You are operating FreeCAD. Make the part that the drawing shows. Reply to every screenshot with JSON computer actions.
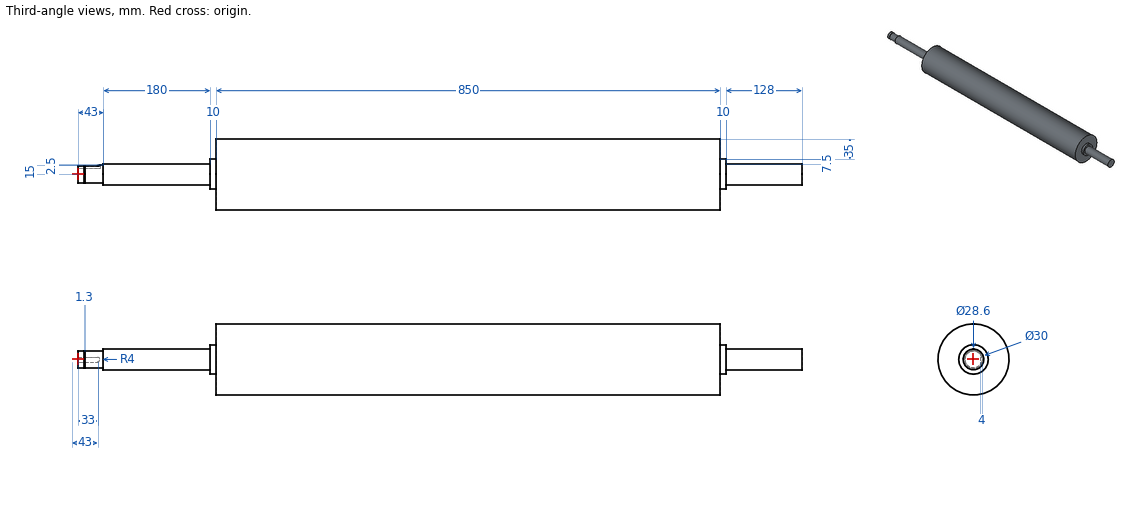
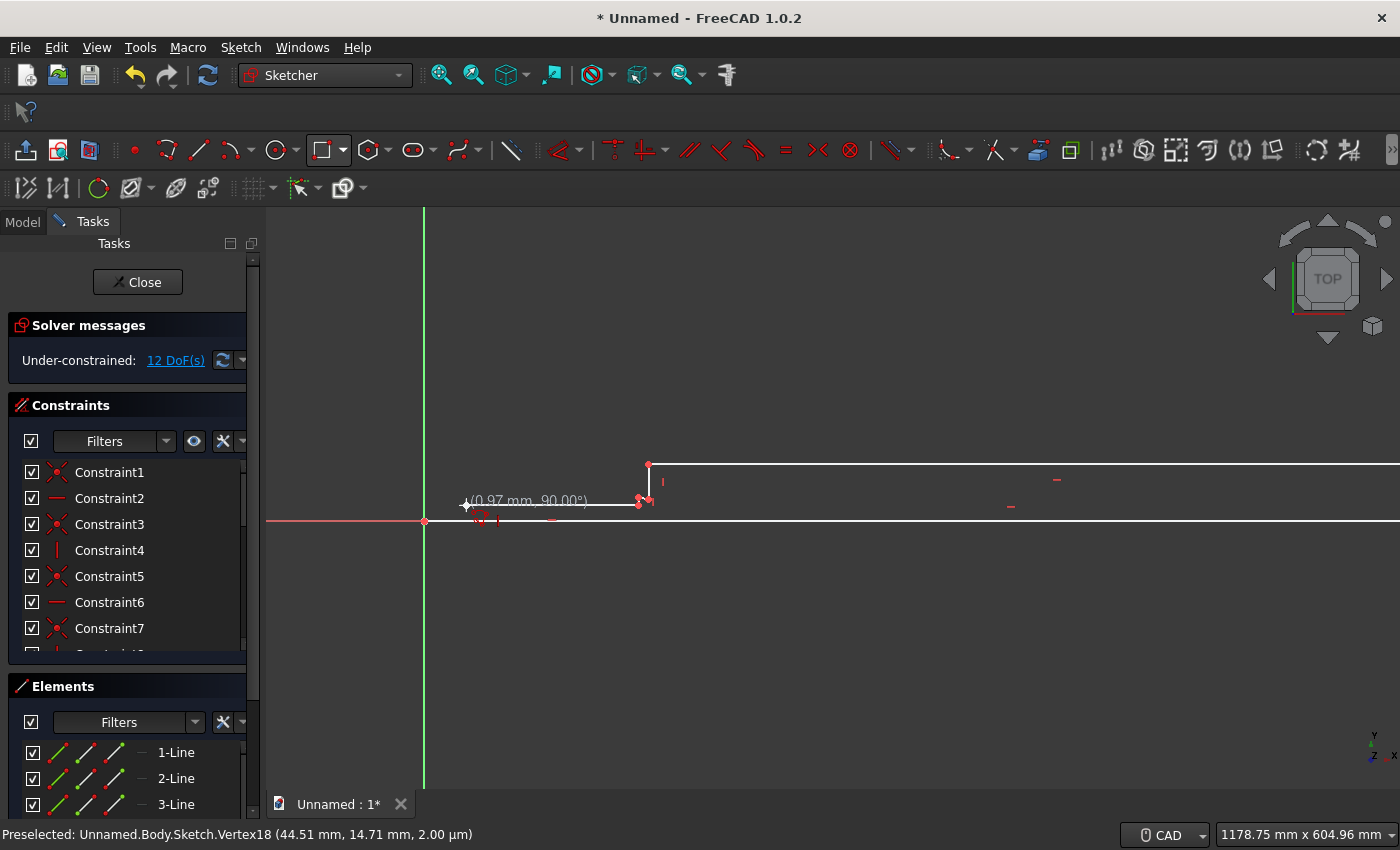
{"action": "scroll", "coordinate": [466, 507], "scroll_direction": "up", "scroll_amount": 10}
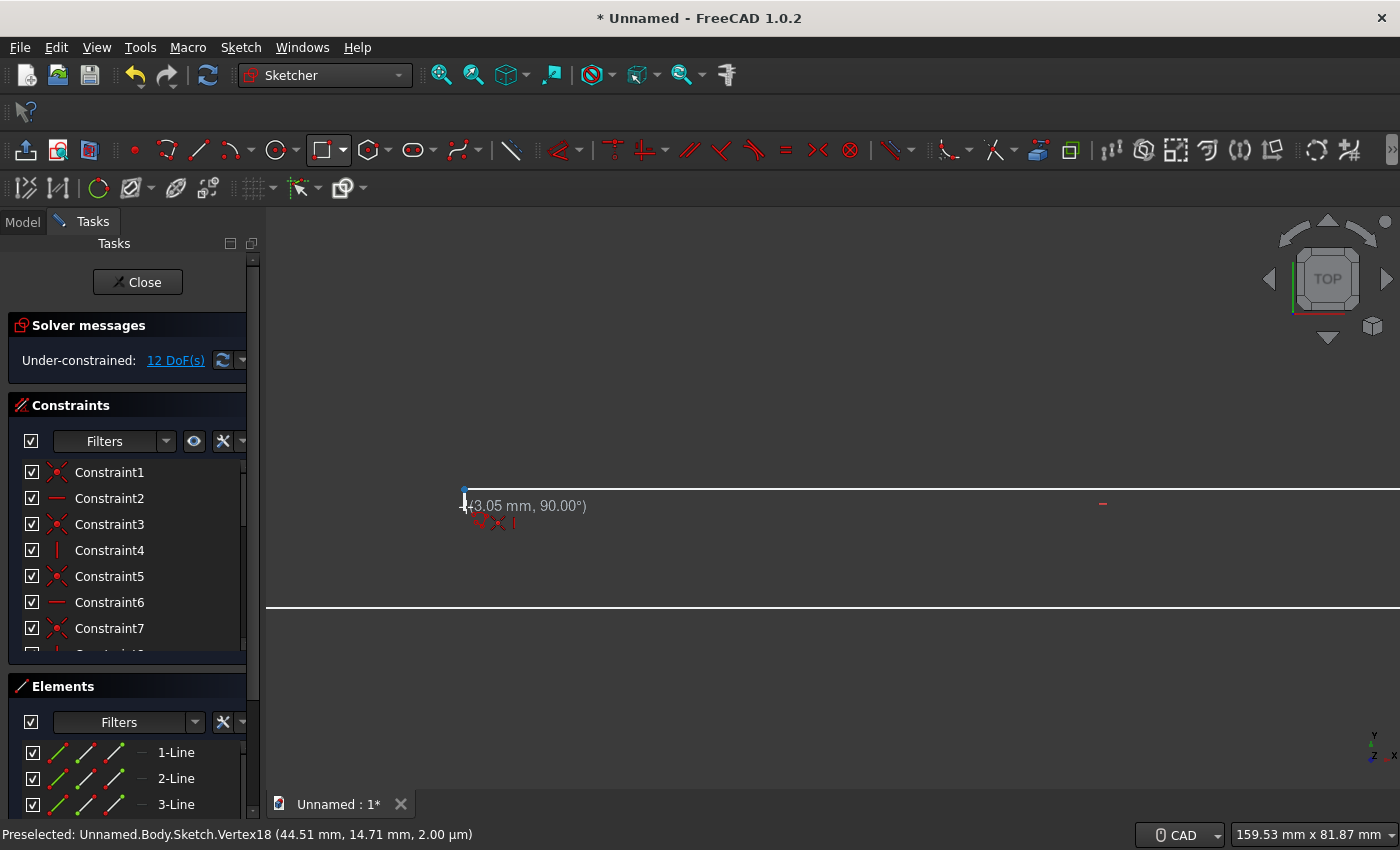
{"action": "left_click", "coordinate": [465, 502]}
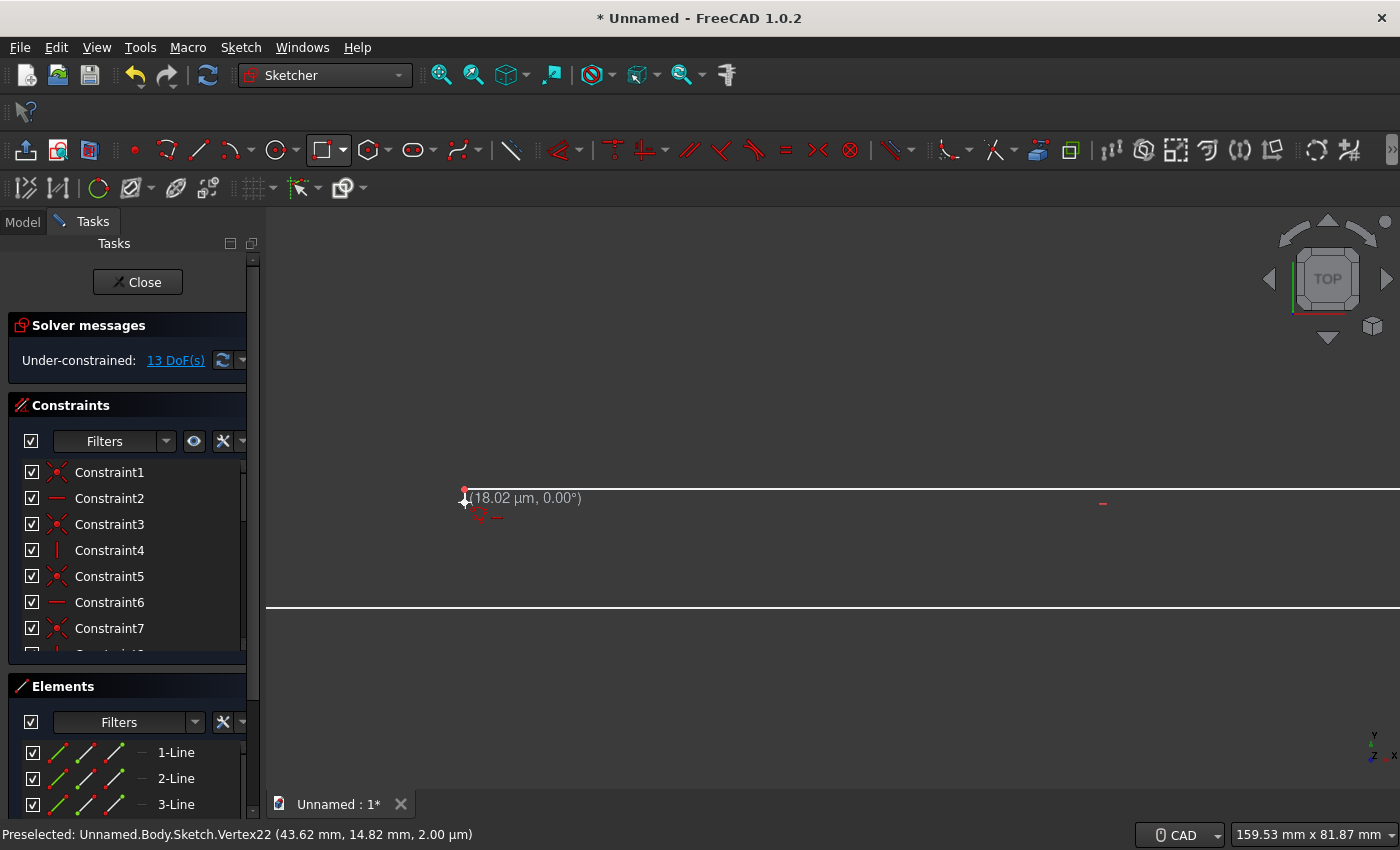
{"action": "scroll", "coordinate": [465, 506], "scroll_direction": "down", "scroll_amount": 13}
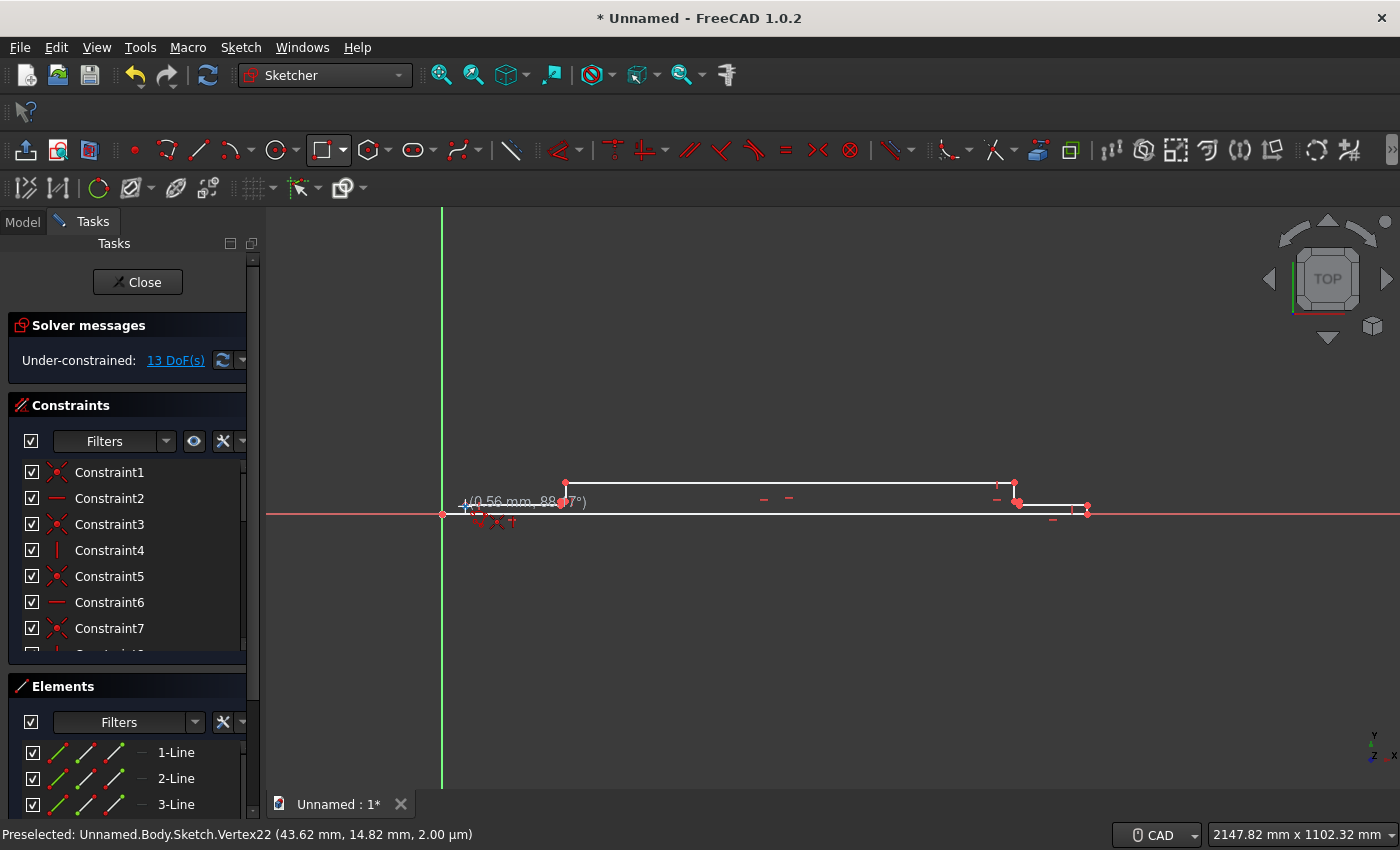
{"action": "scroll", "coordinate": [442, 506], "scroll_direction": "up", "scroll_amount": 4}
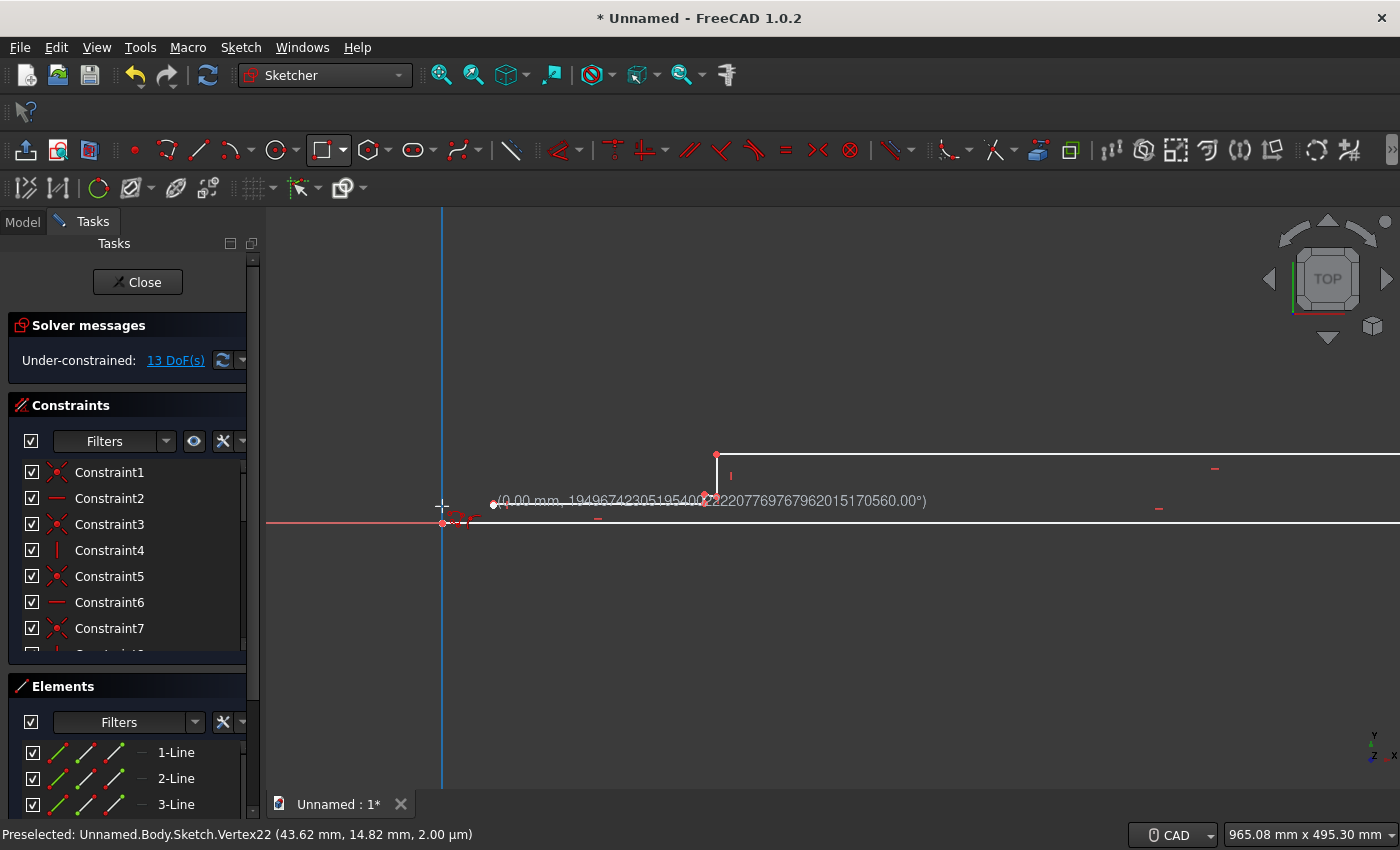
{"action": "left_click", "coordinate": [451, 506]}
{"action": "left_click", "coordinate": [442, 523]}
{"action": "key", "text": "Escape"}
{"action": "key", "text": "Escape"}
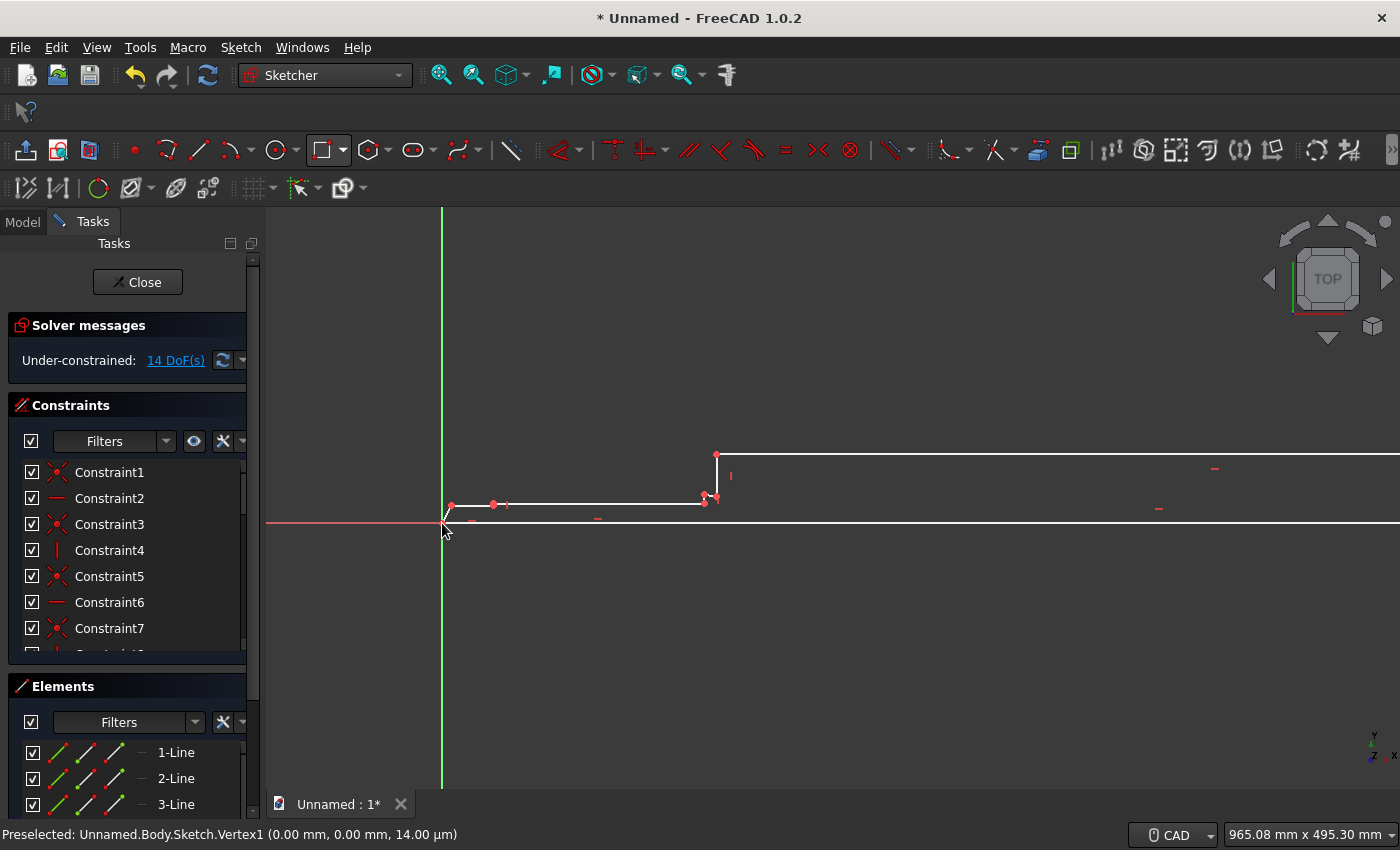
{"action": "scroll", "coordinate": [711, 496], "scroll_direction": "up", "scroll_amount": 5}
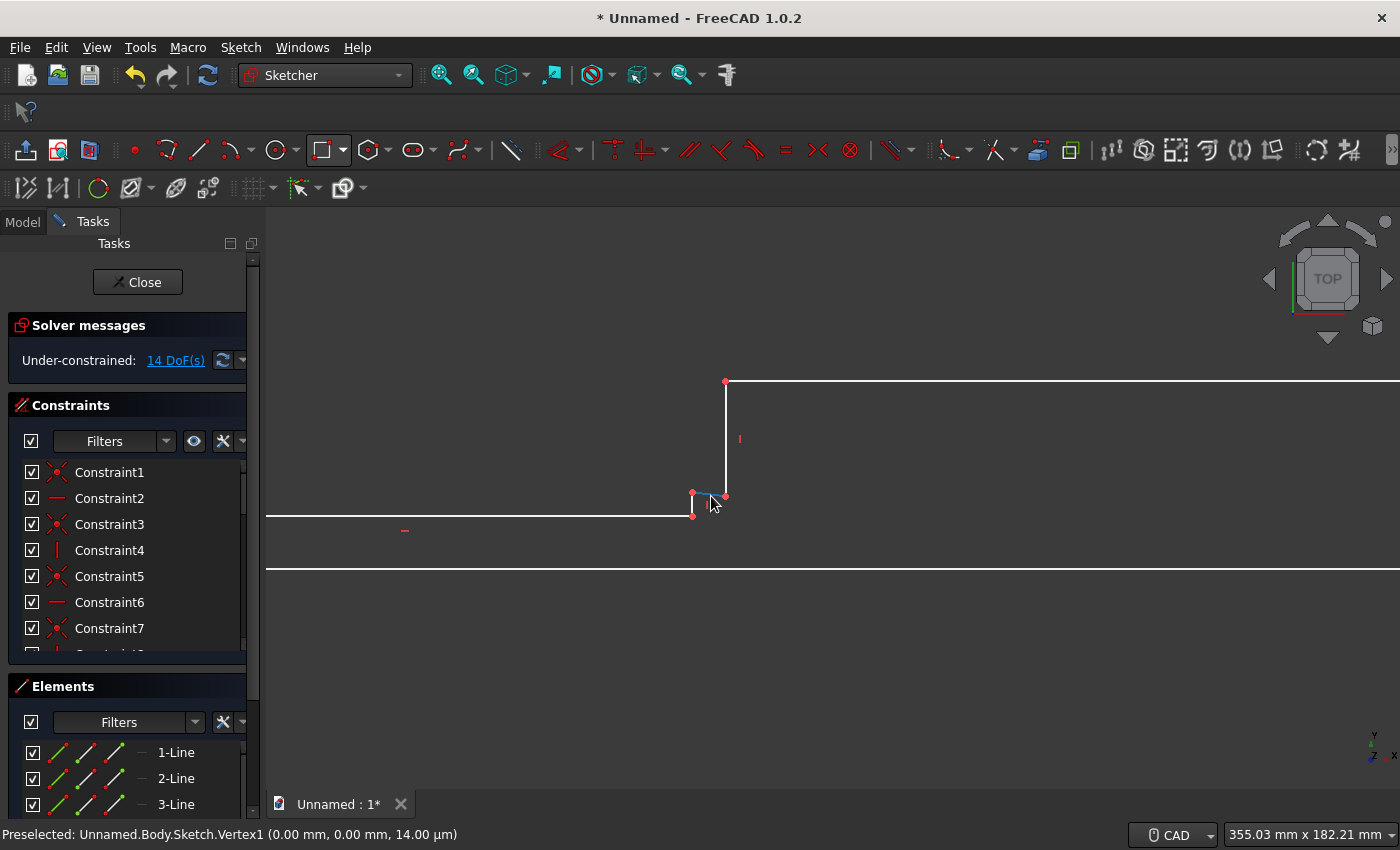
{"action": "left_click", "coordinate": [709, 494]}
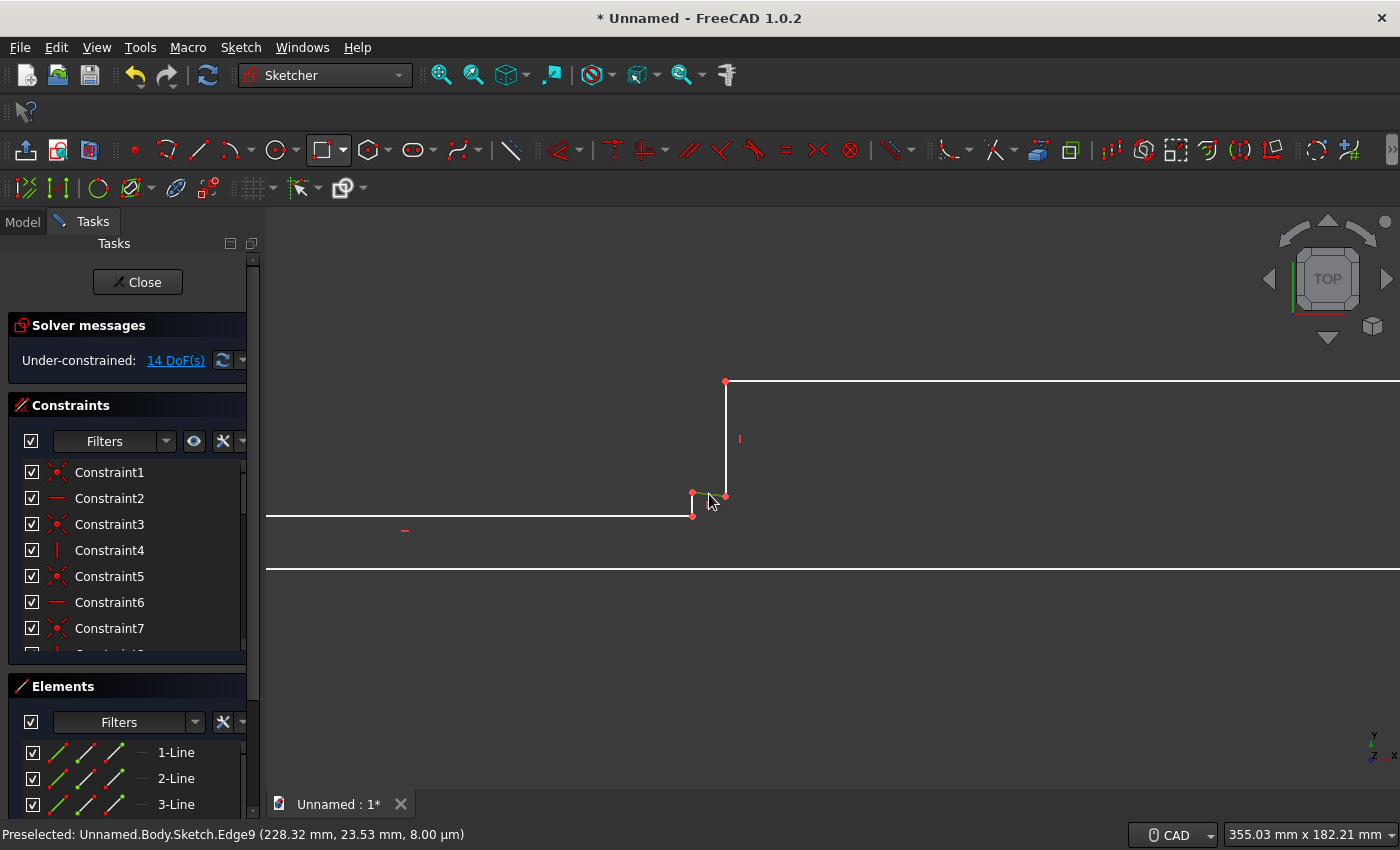
{"action": "left_click", "coordinate": [668, 150]}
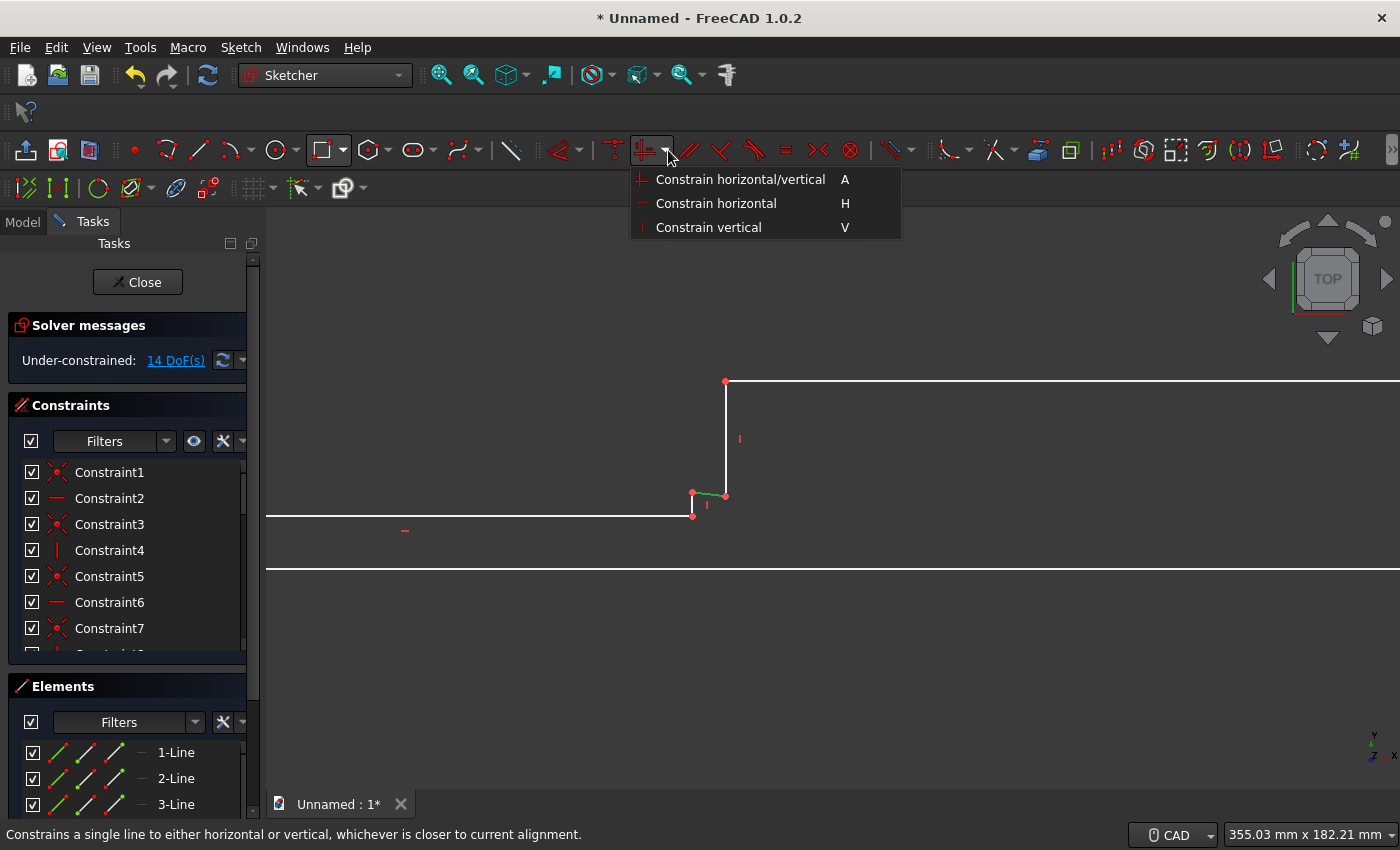
{"action": "left_click", "coordinate": [766, 203]}